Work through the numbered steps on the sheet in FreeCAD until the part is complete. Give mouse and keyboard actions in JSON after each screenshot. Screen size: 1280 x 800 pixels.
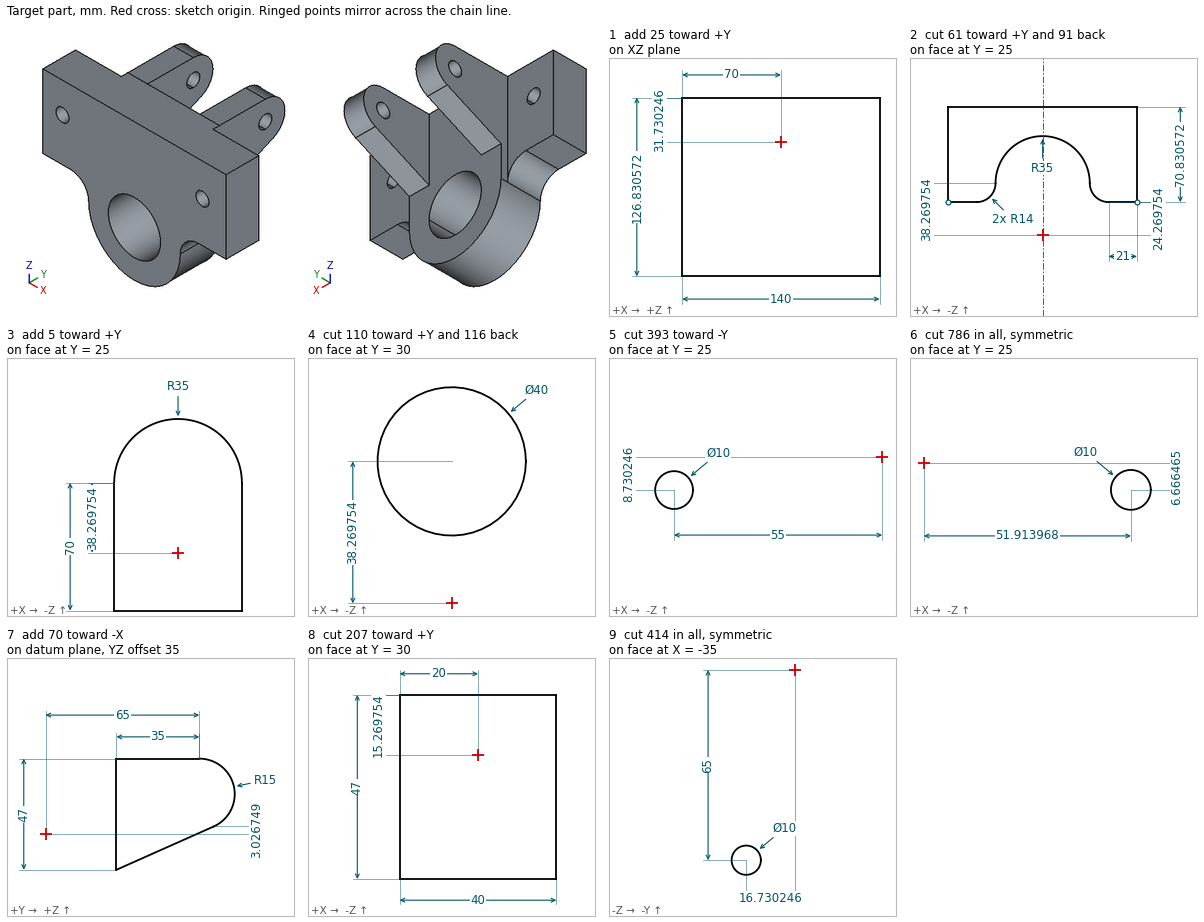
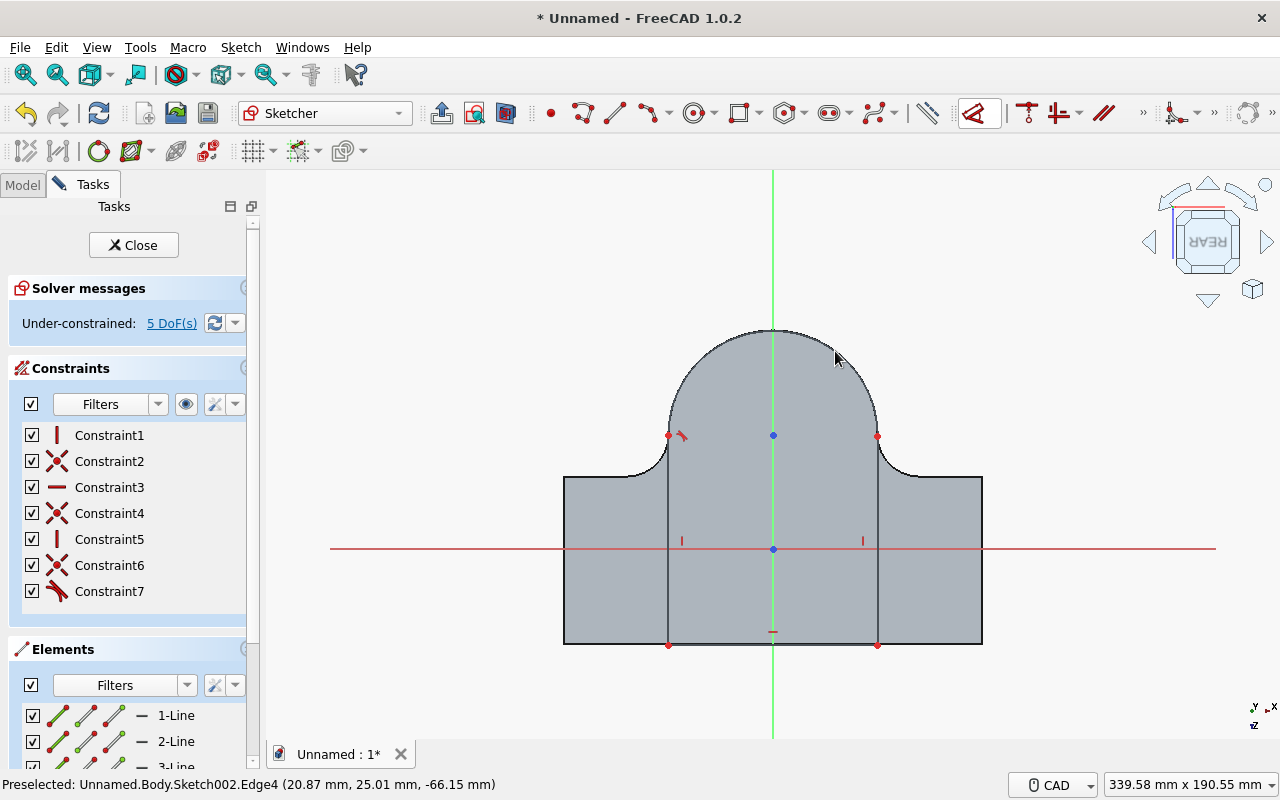
{"action": "left_click", "coordinate": [878, 583]}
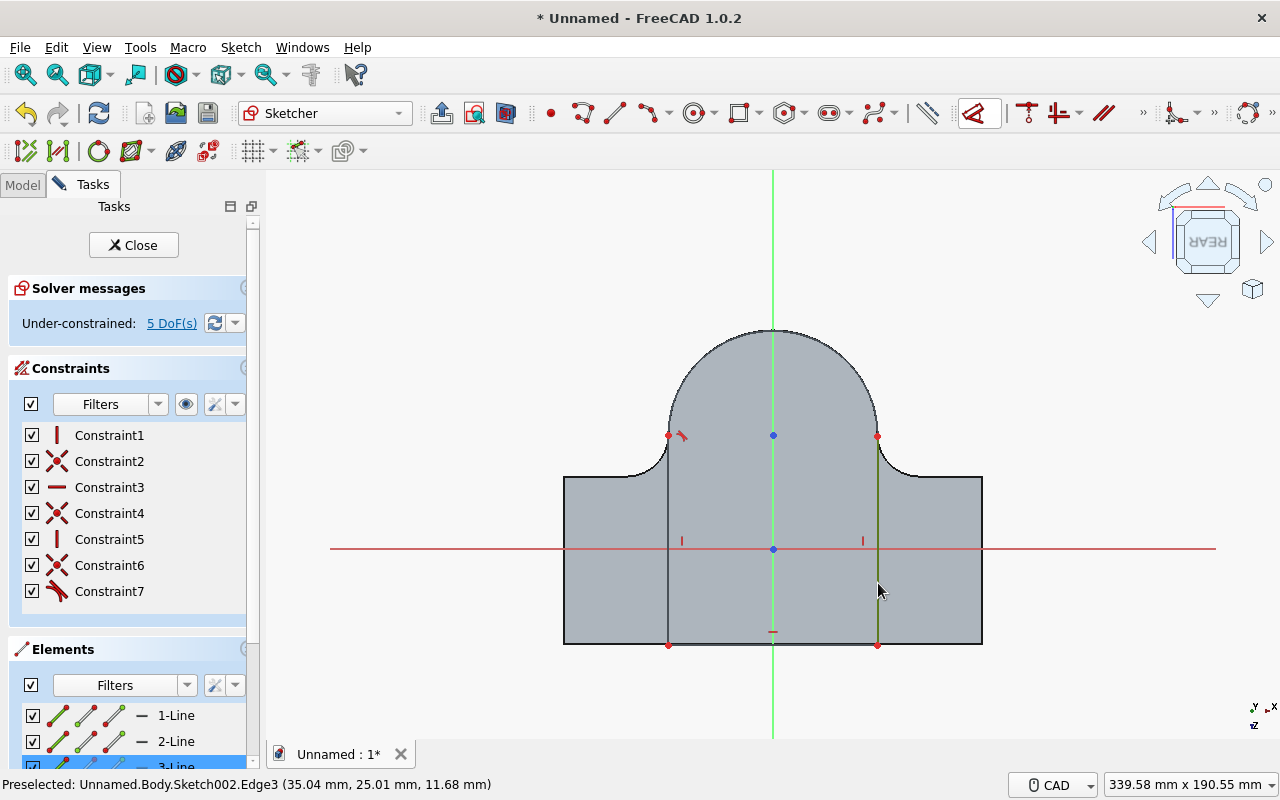
{"action": "left_click", "coordinate": [835, 351]}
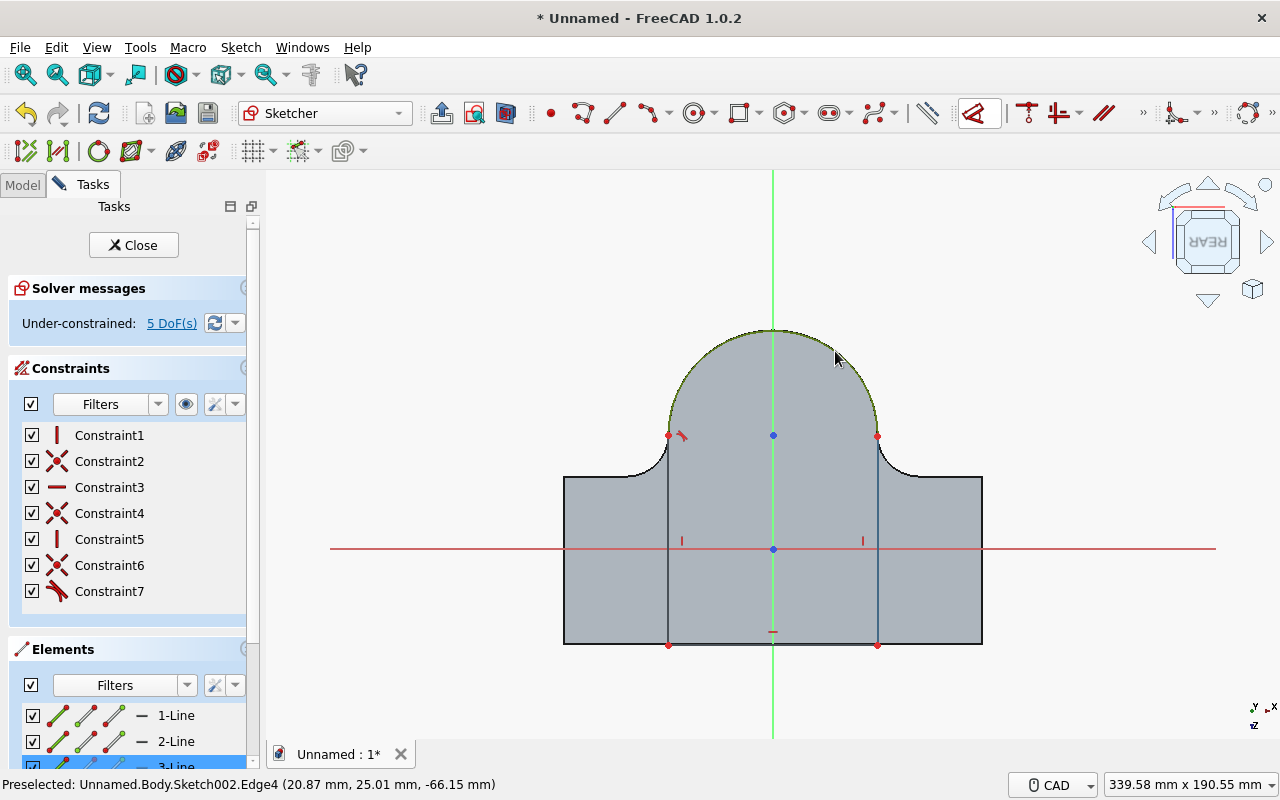
{"action": "key", "text": "t"}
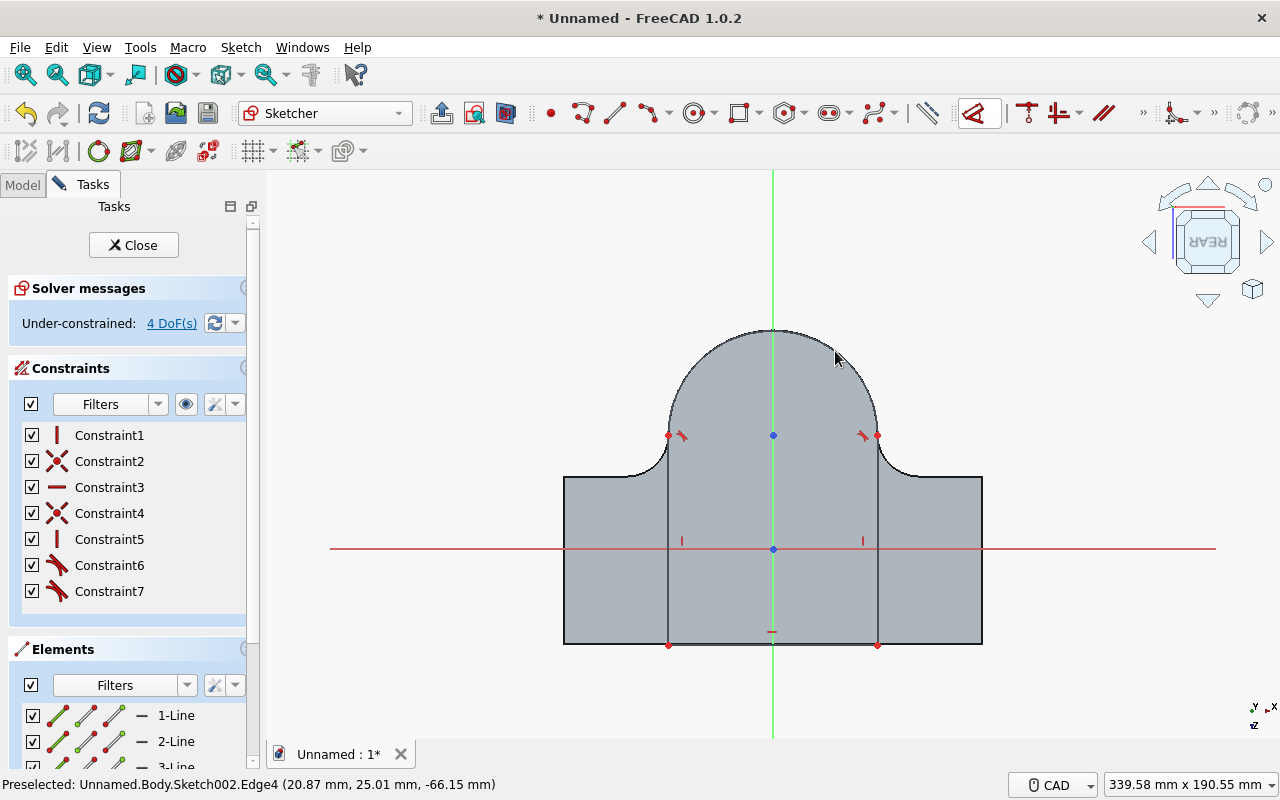
{"action": "left_click", "coordinate": [773, 436]}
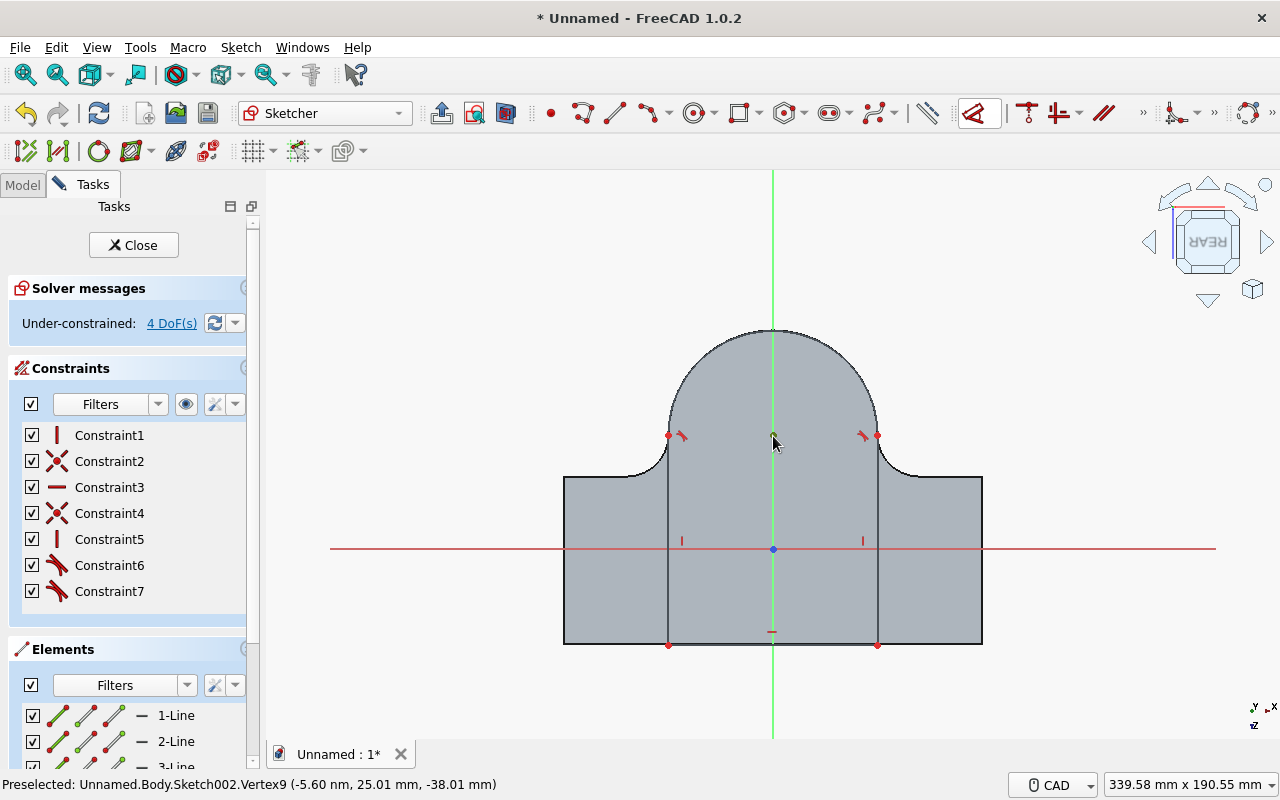
{"action": "left_click", "coordinate": [773, 601]}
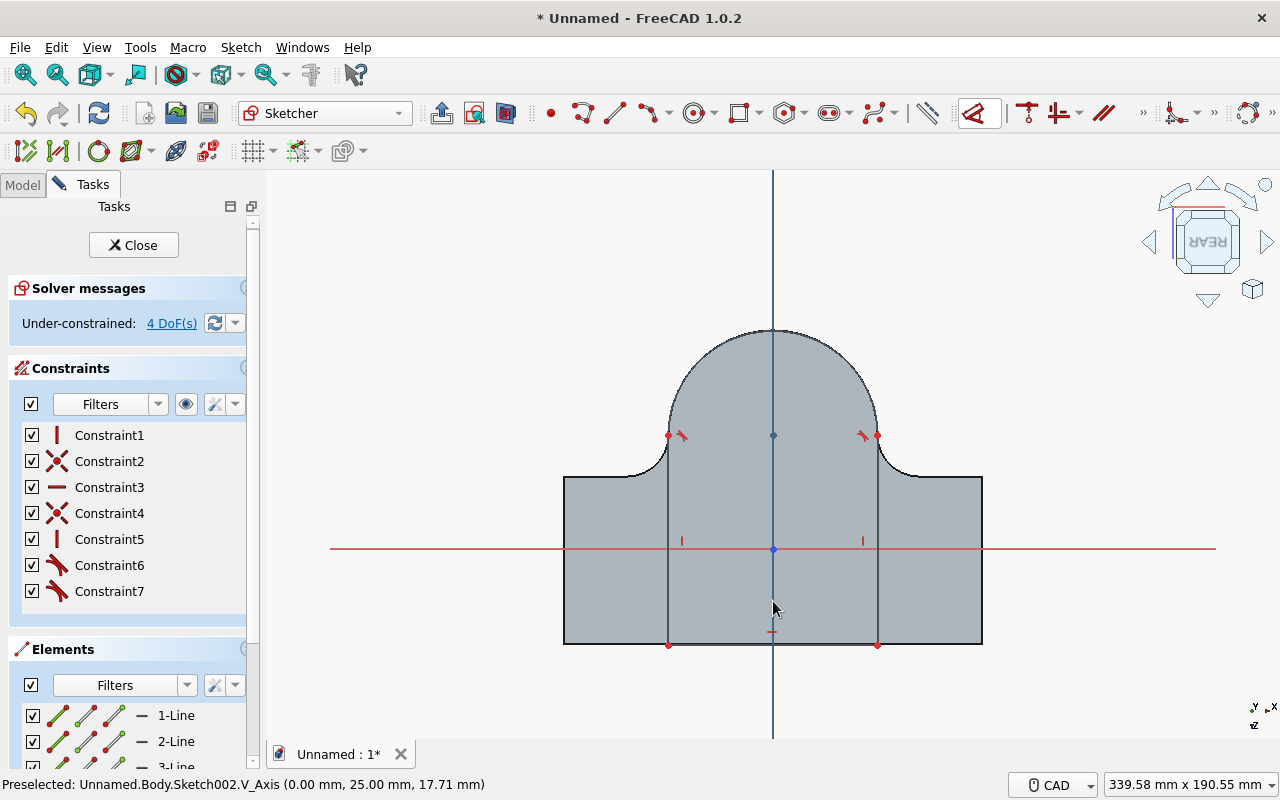
{"action": "left_click", "coordinate": [1028, 114]}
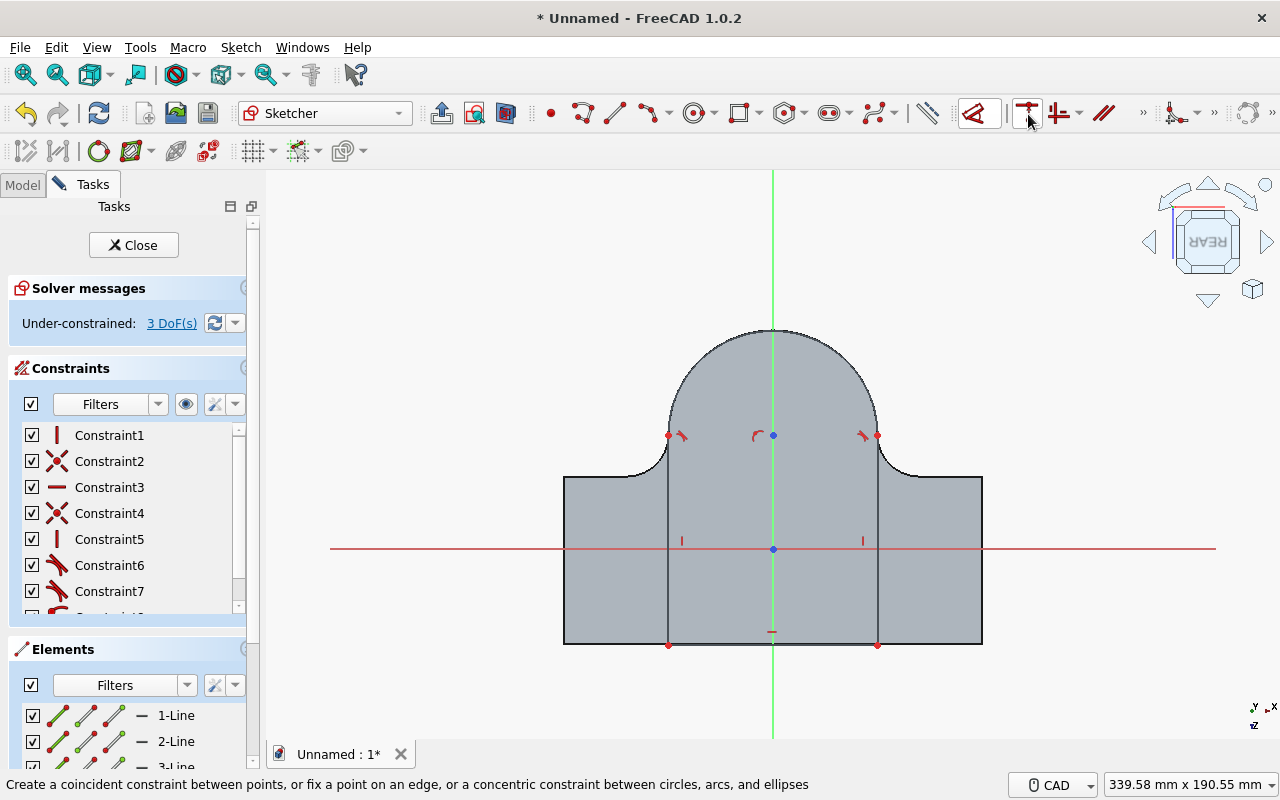
{"action": "left_click", "coordinate": [835, 351]}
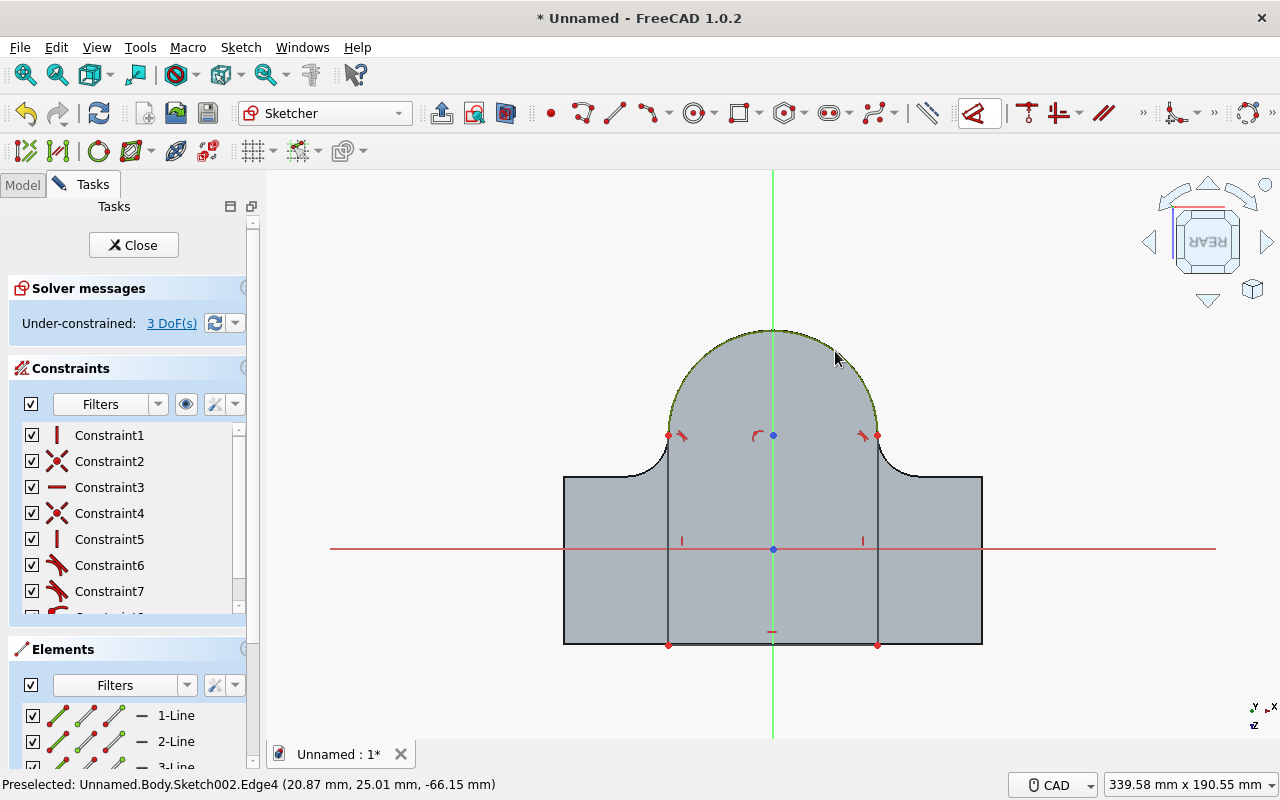
{"action": "left_click", "coordinate": [996, 114]}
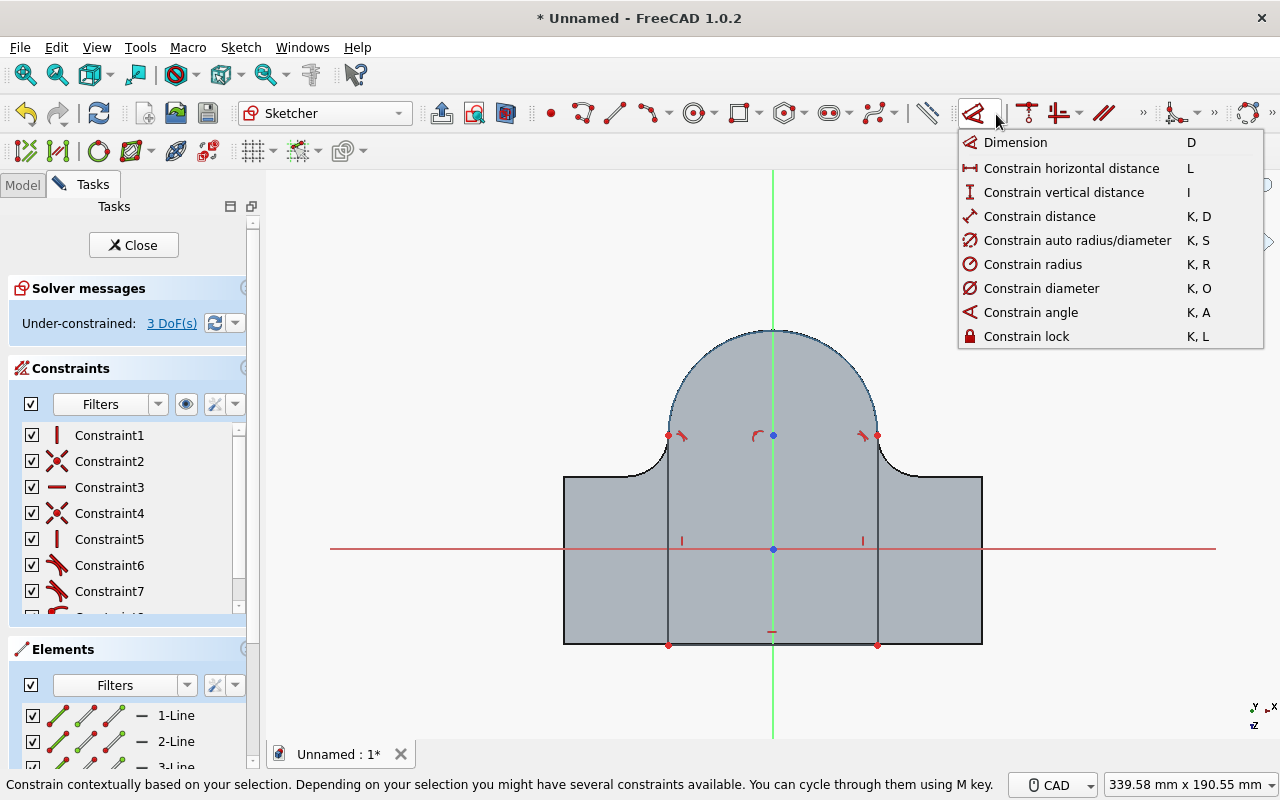
{"action": "left_click", "coordinate": [1111, 264]}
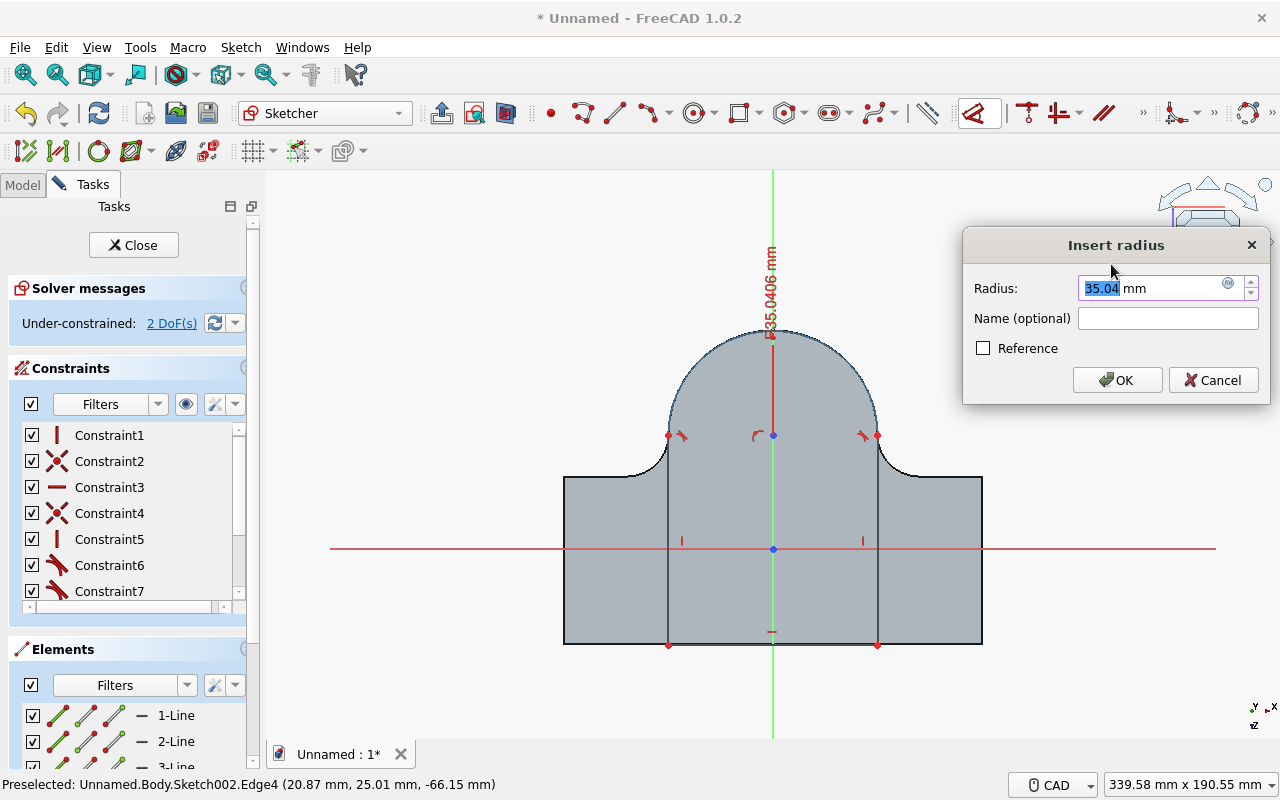
{"action": "type", "text": "35"}
{"action": "key", "text": "Return"}